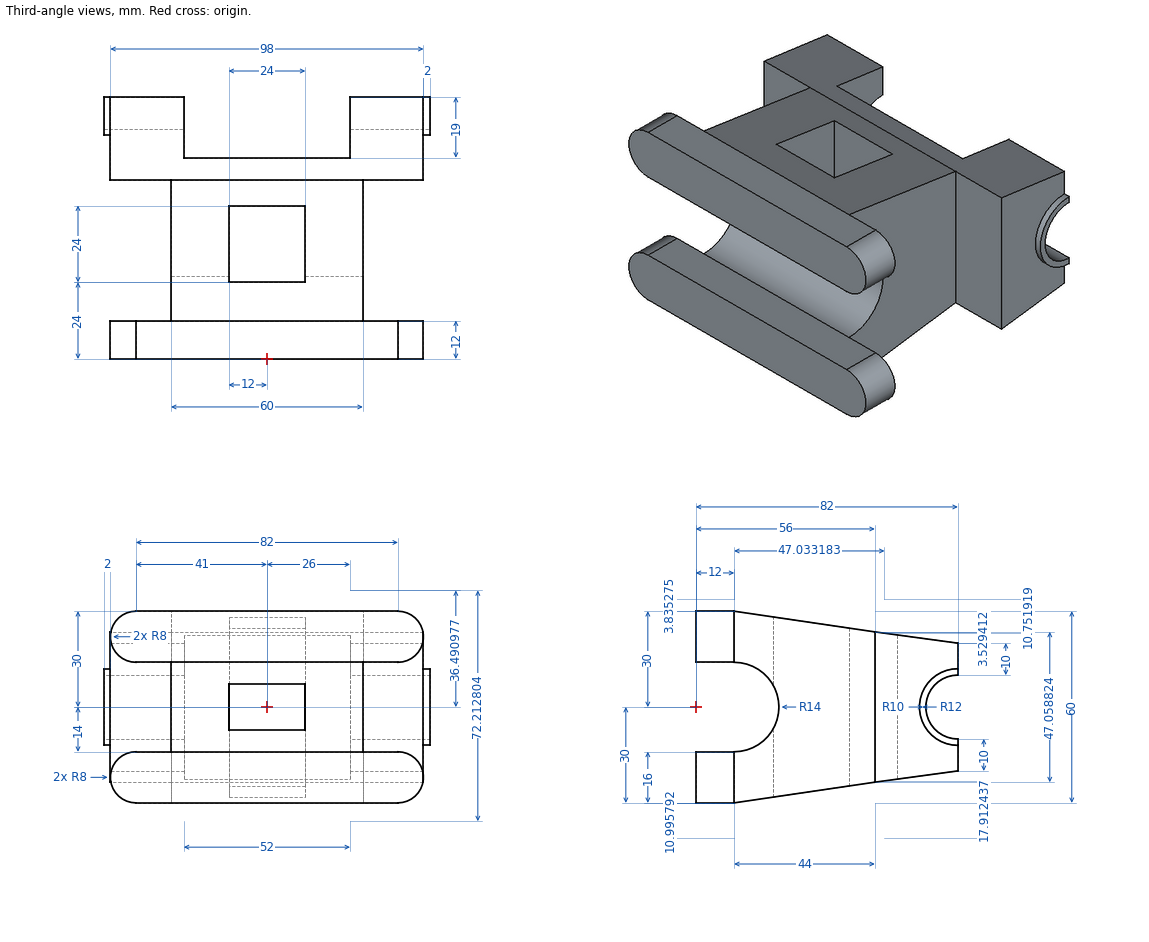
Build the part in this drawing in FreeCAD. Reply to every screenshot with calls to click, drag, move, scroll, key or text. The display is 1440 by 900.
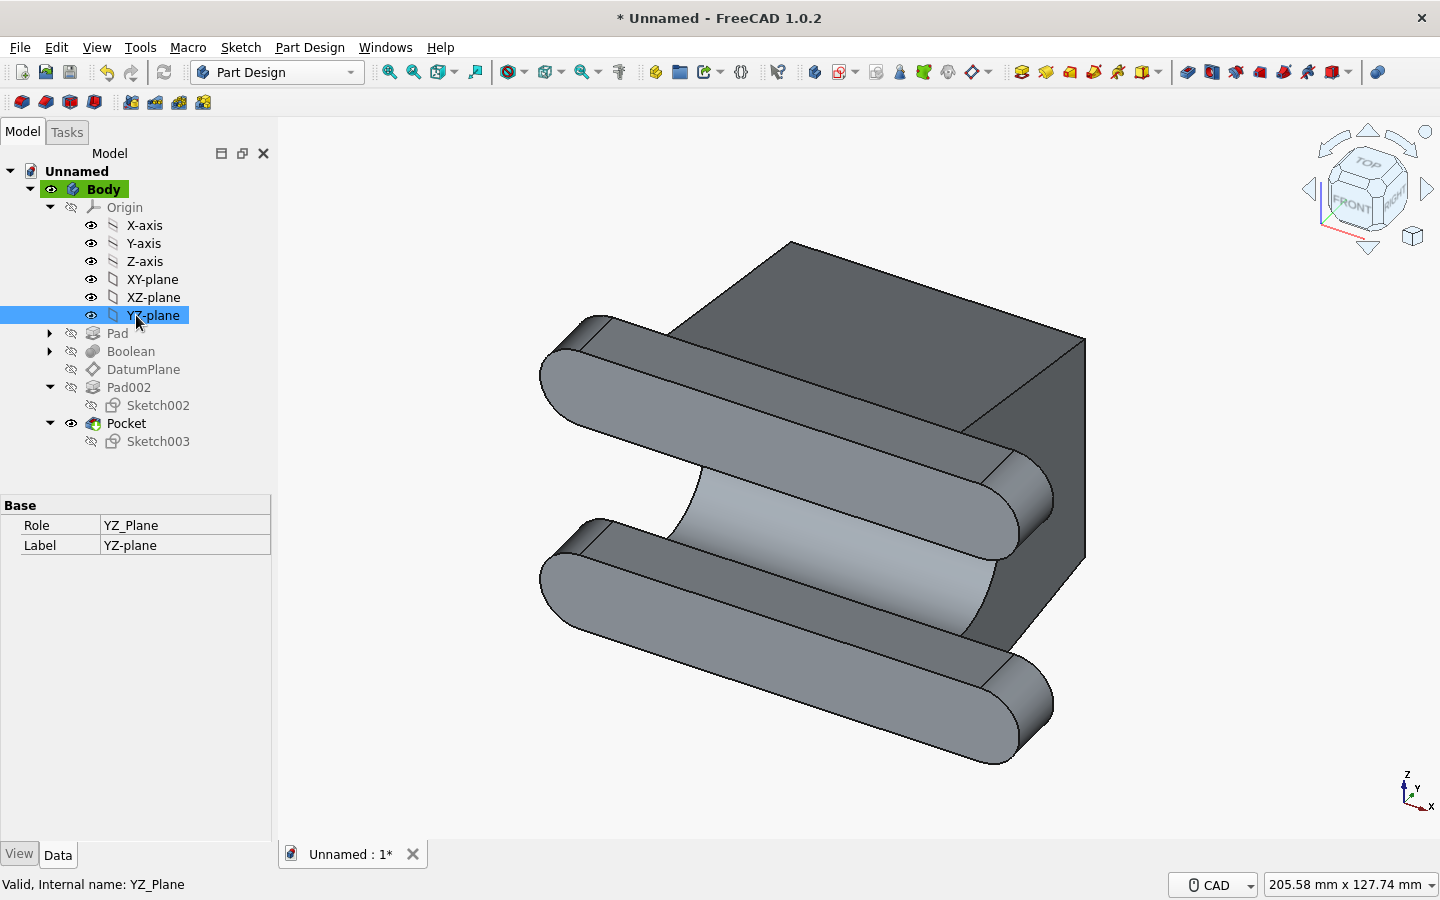
click(972, 72)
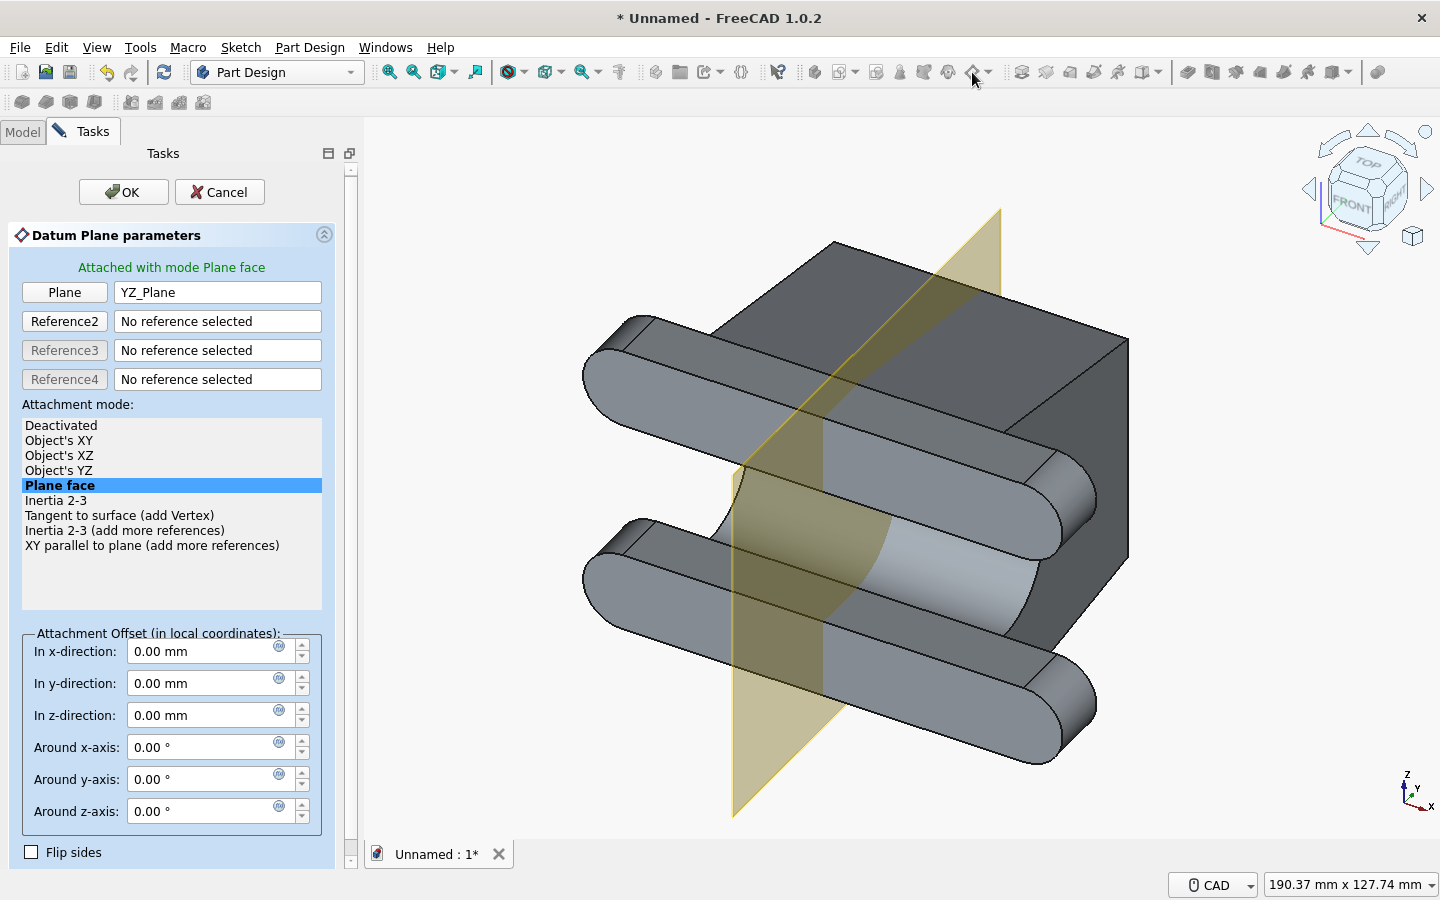
triple_click(210, 715)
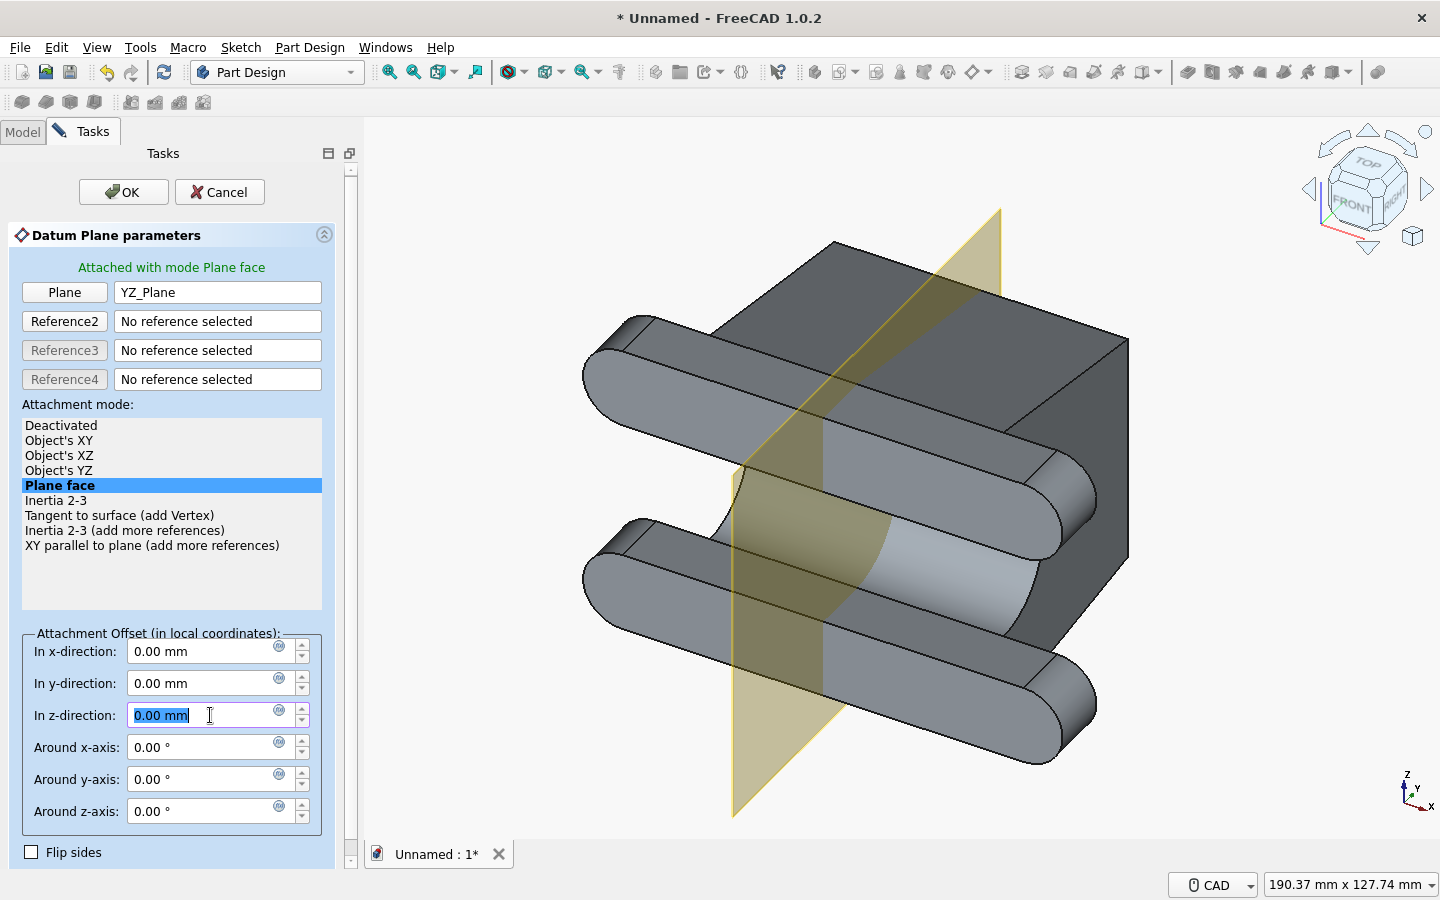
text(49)
key(Tab)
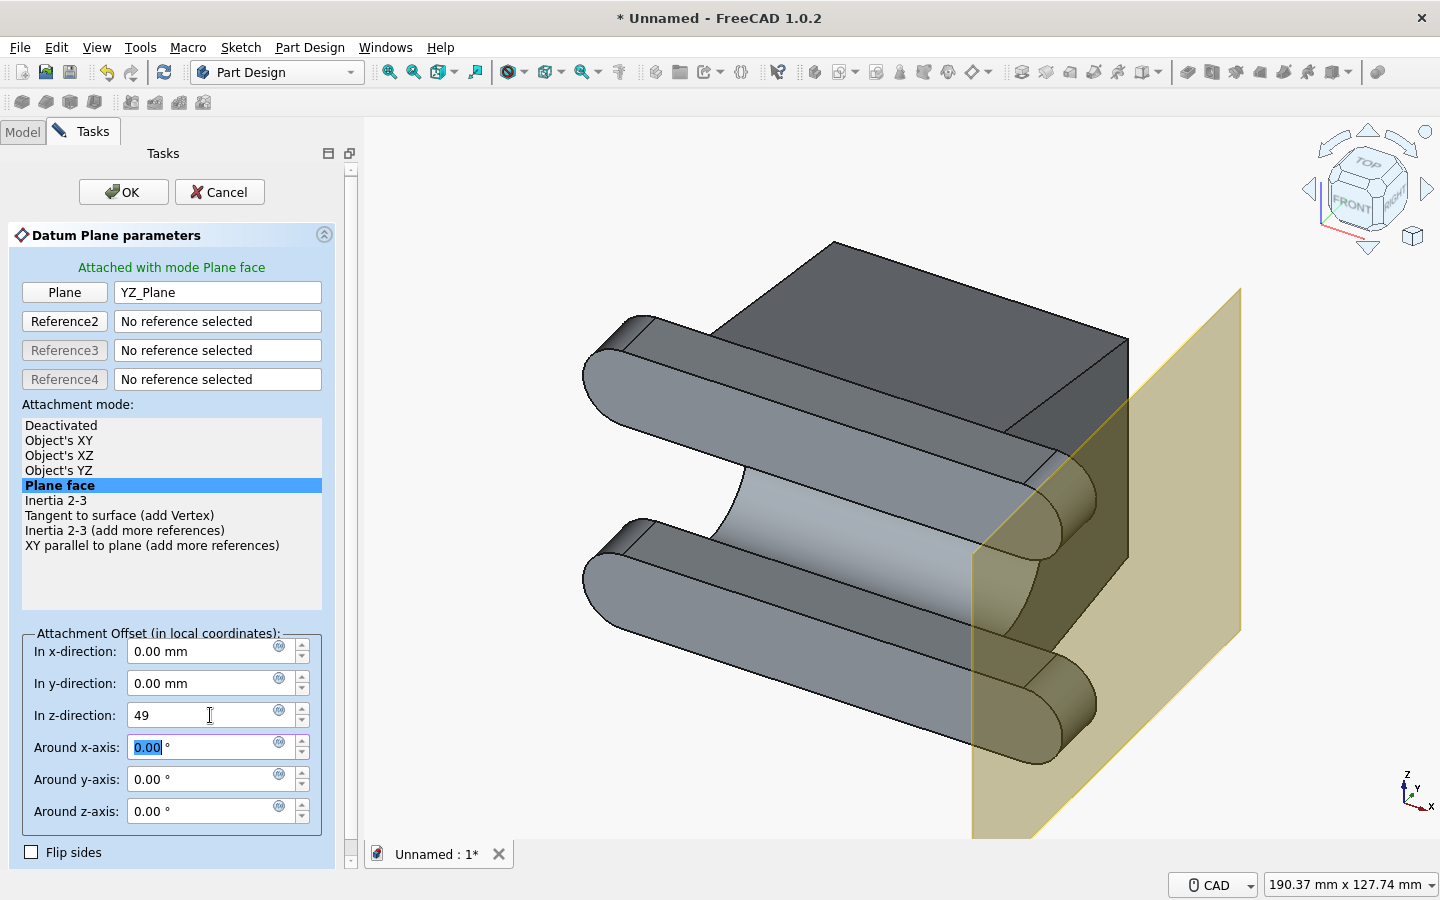
click(124, 192)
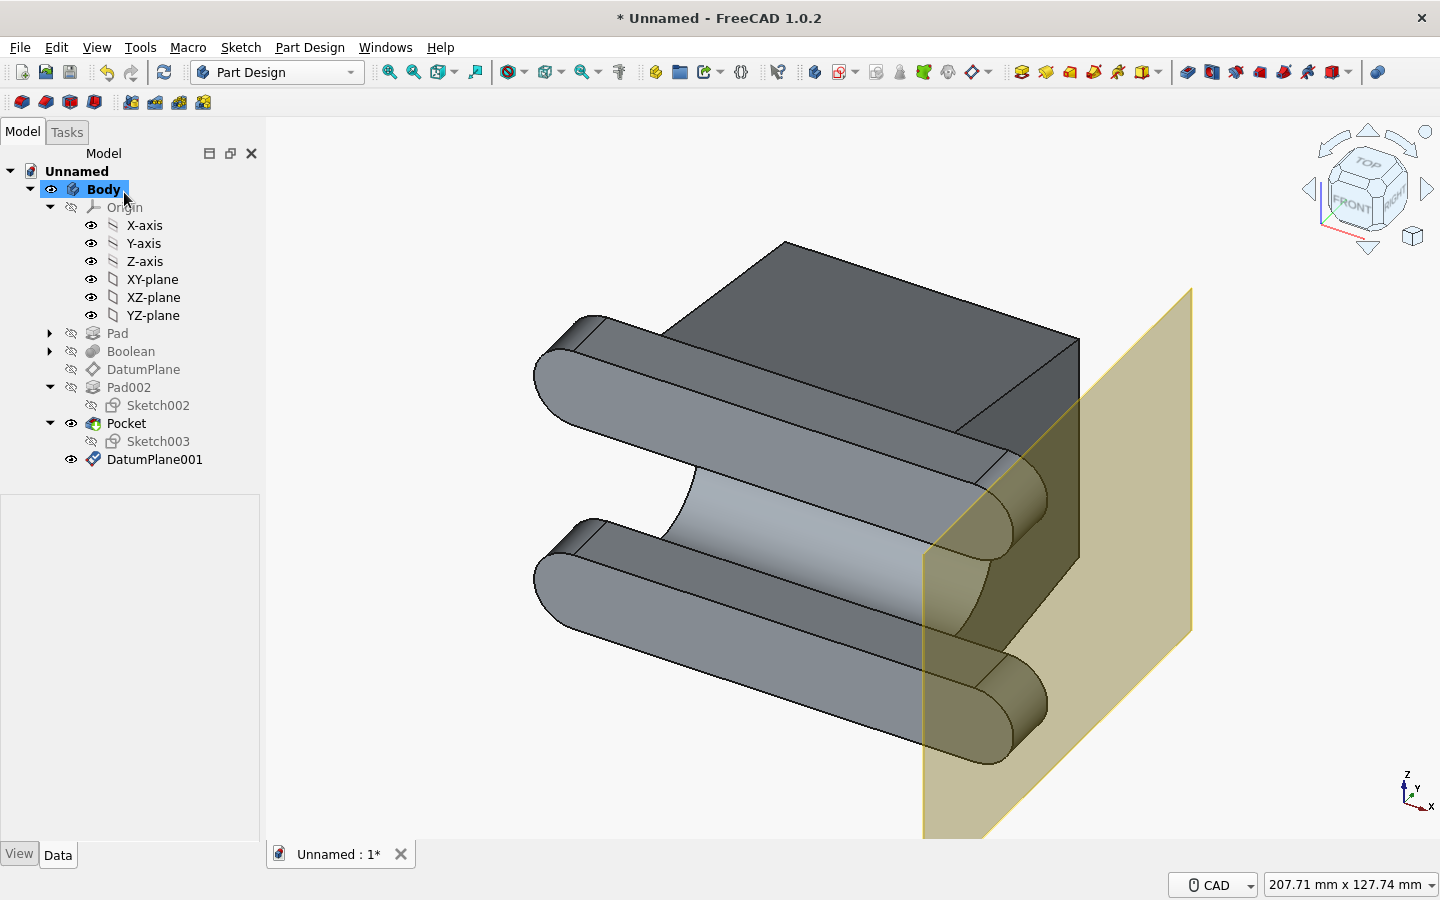
click(116, 459)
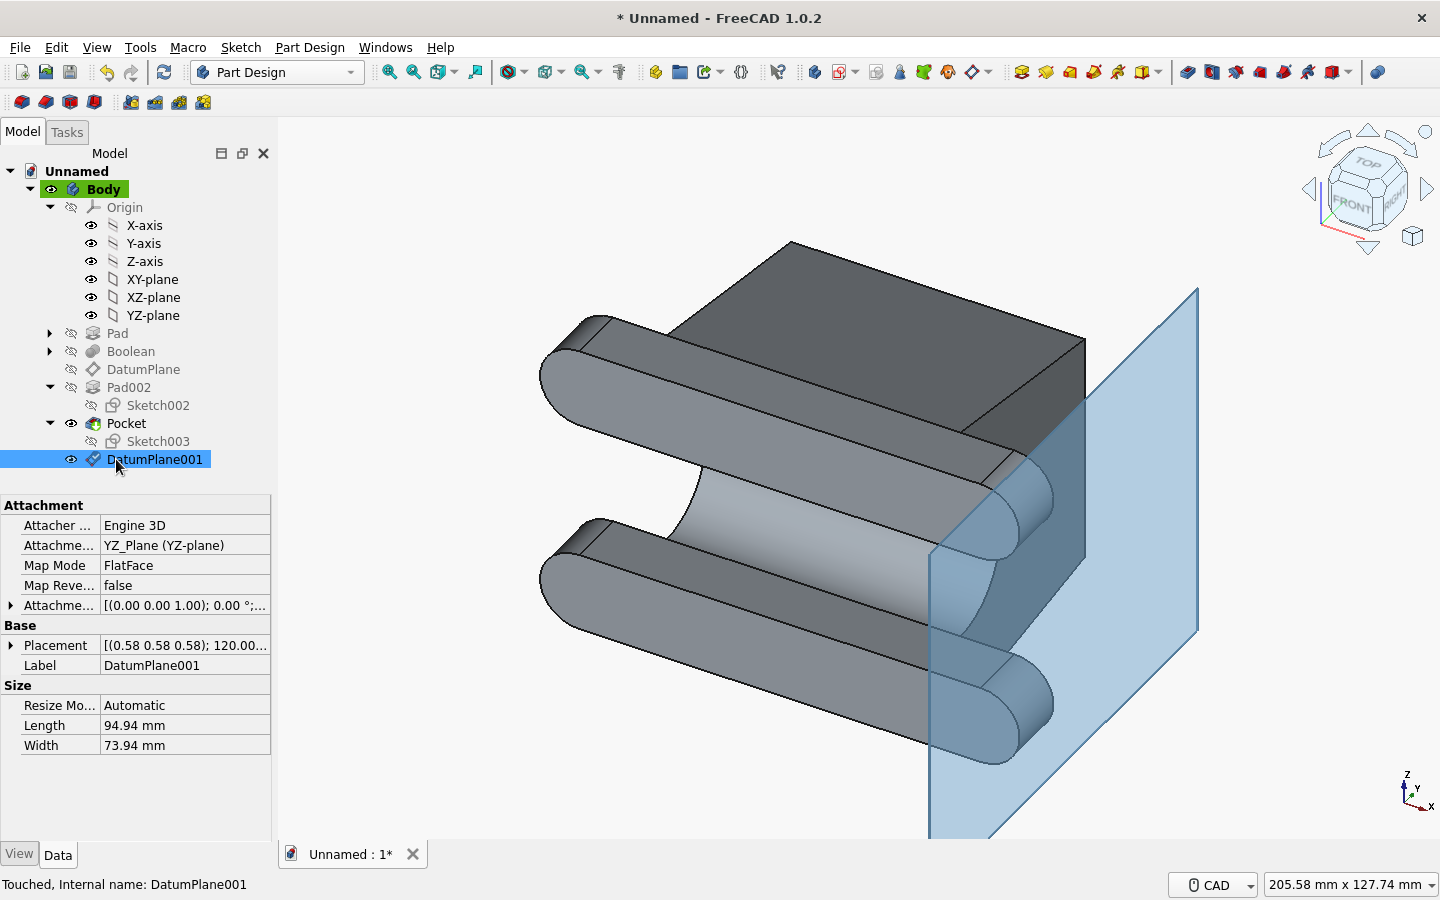
click(840, 72)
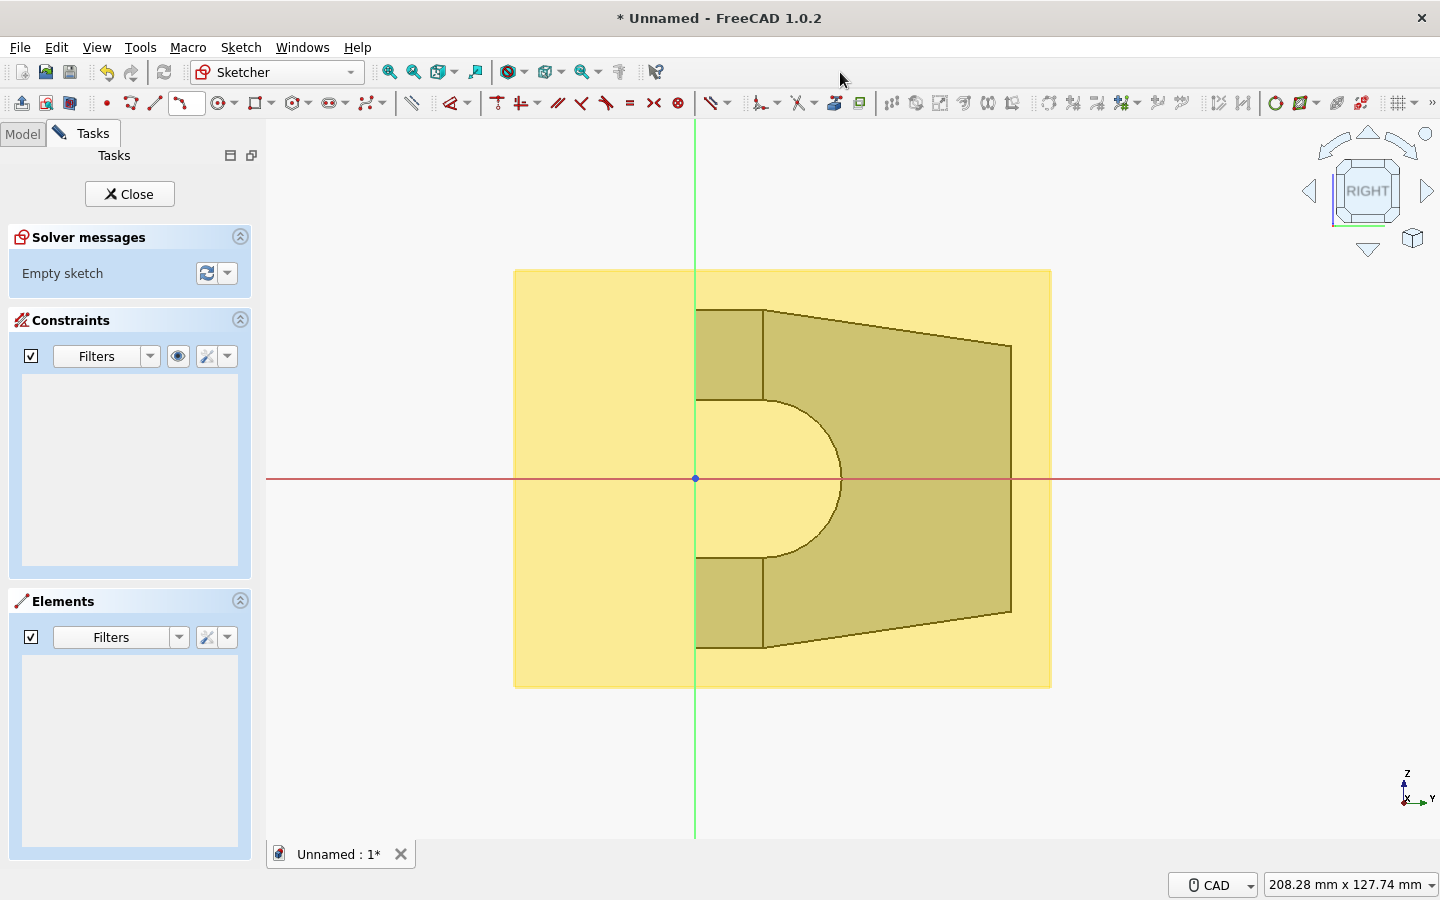
scroll(1215, 479, up, 2)